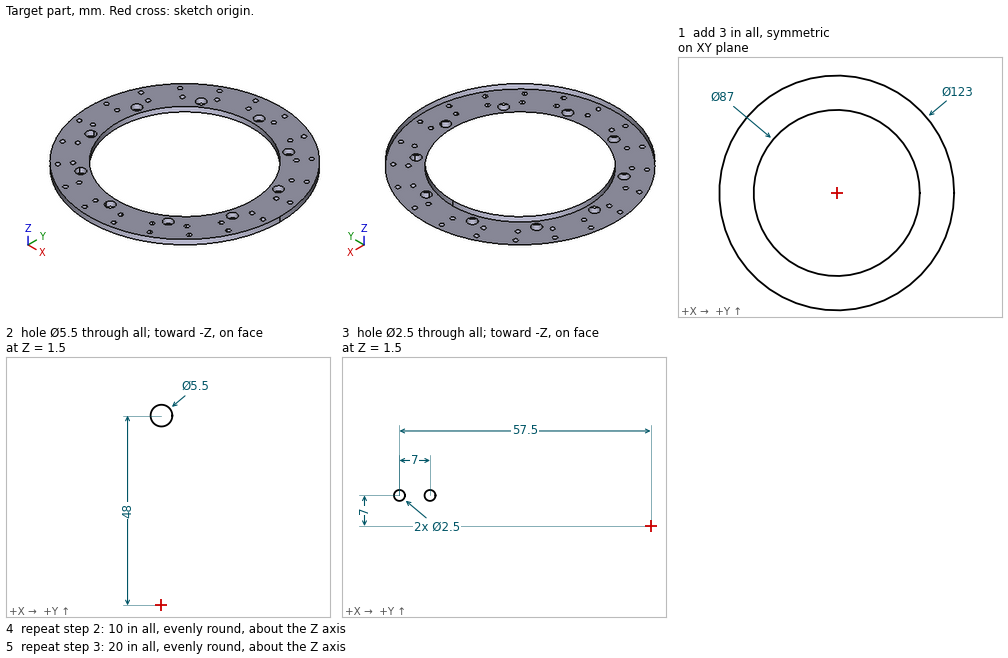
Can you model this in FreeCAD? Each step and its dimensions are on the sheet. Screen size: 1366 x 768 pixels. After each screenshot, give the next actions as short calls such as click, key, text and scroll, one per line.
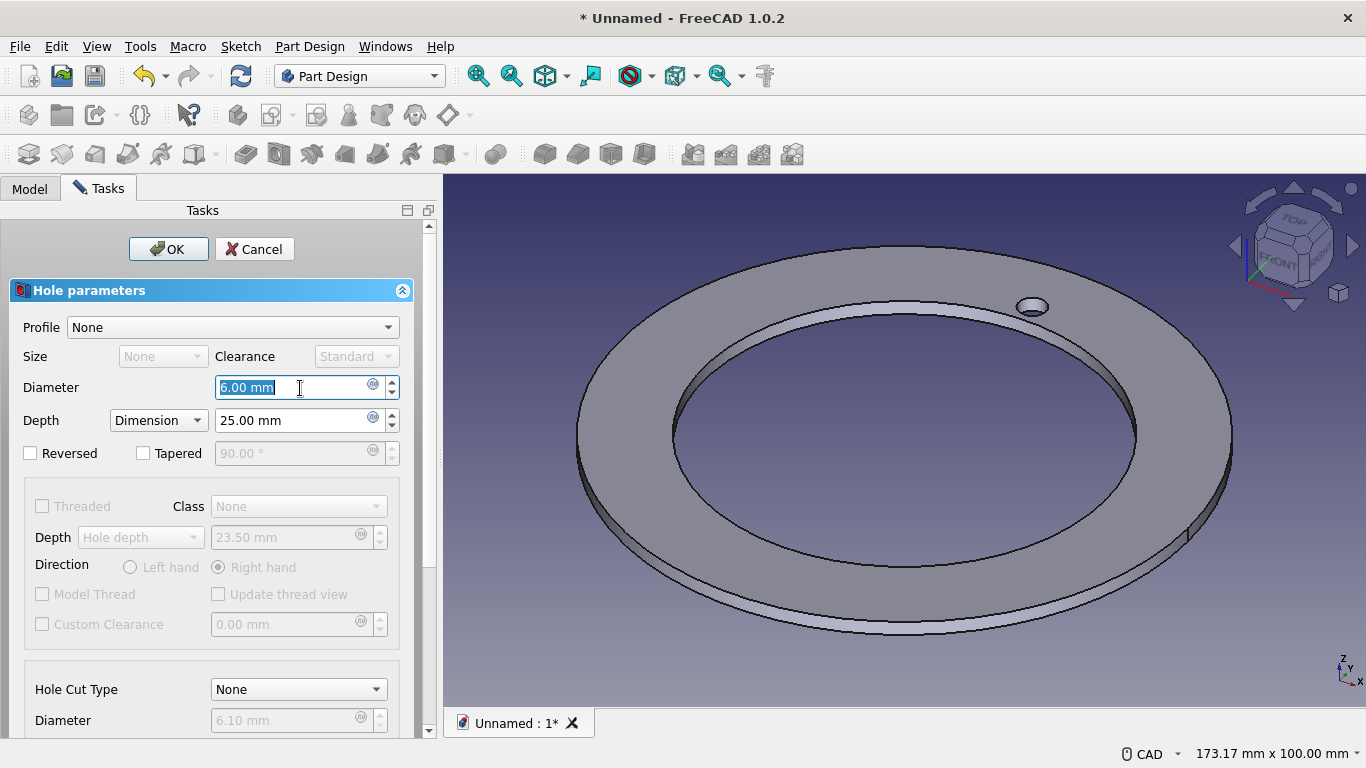
text(5.5)
key(Tab)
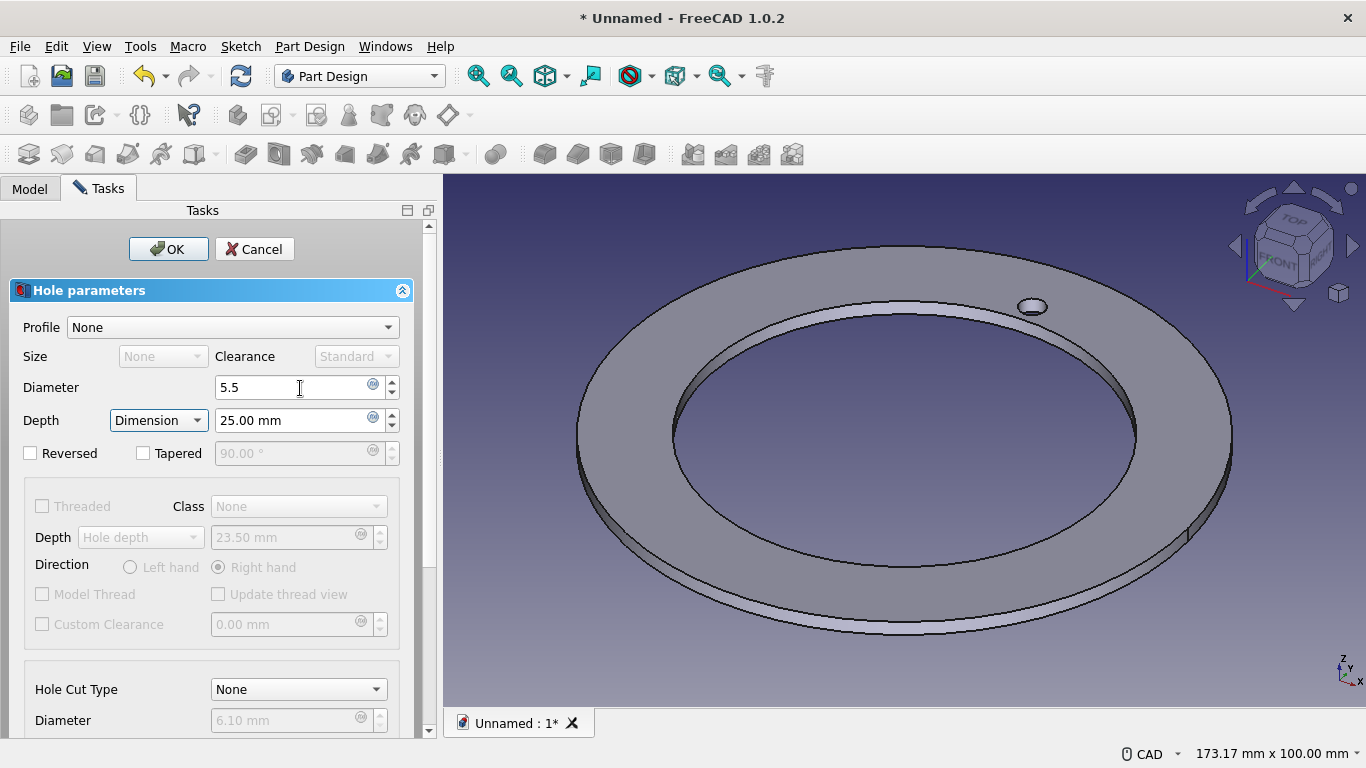
click(160, 420)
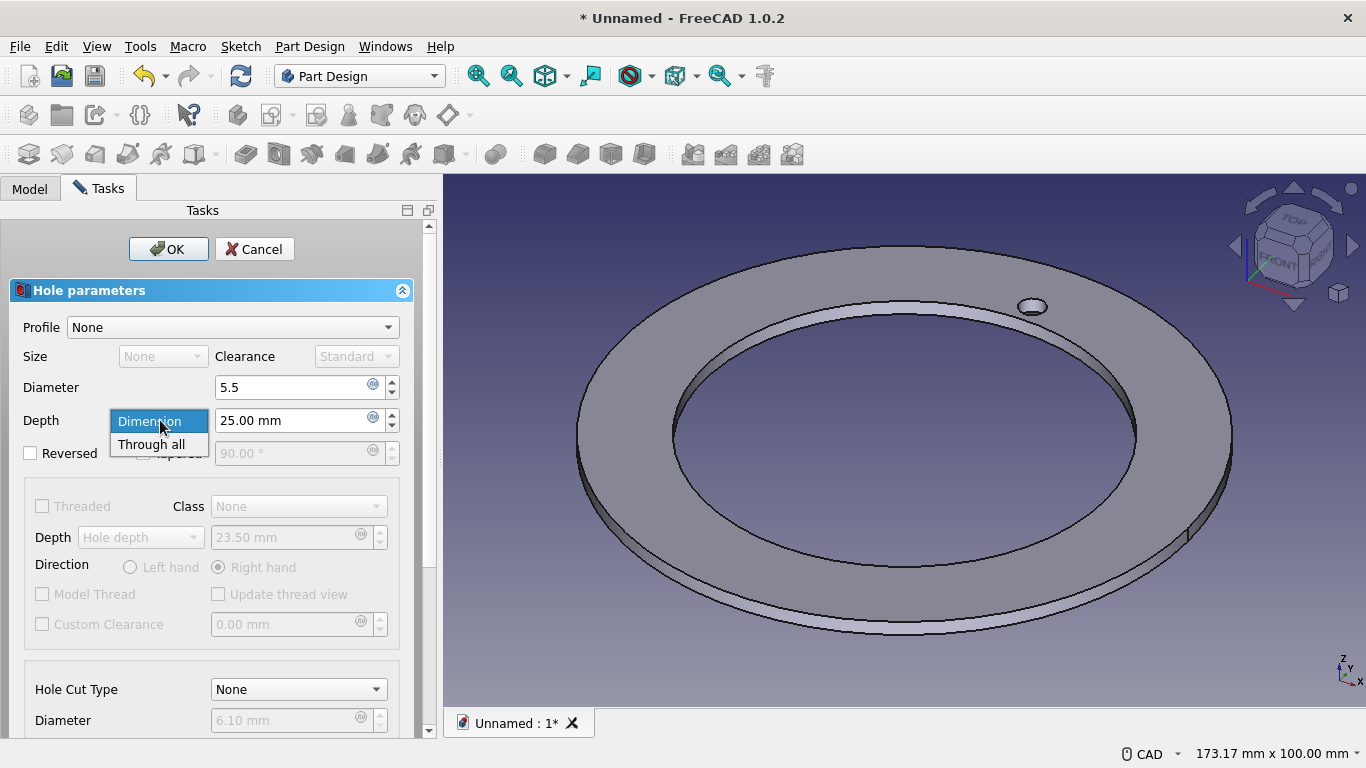
click(158, 444)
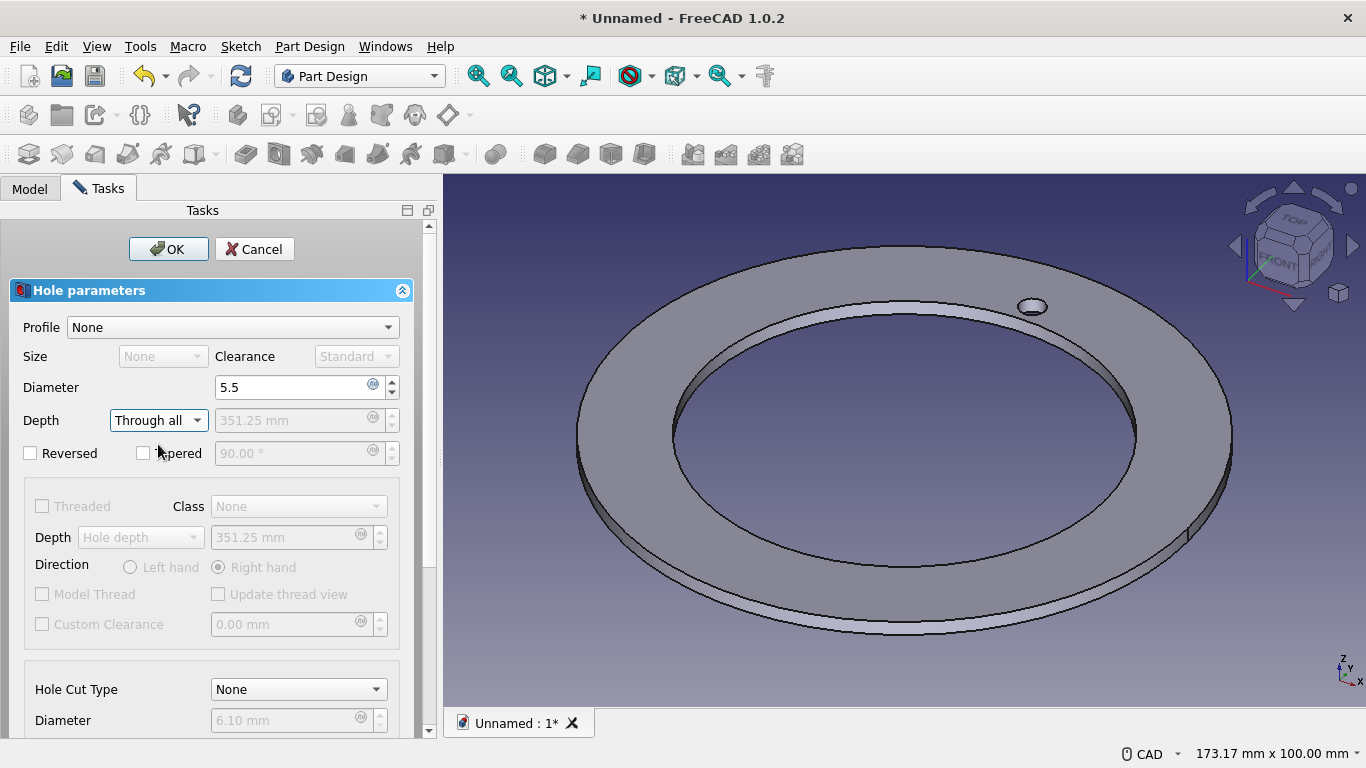
click(169, 249)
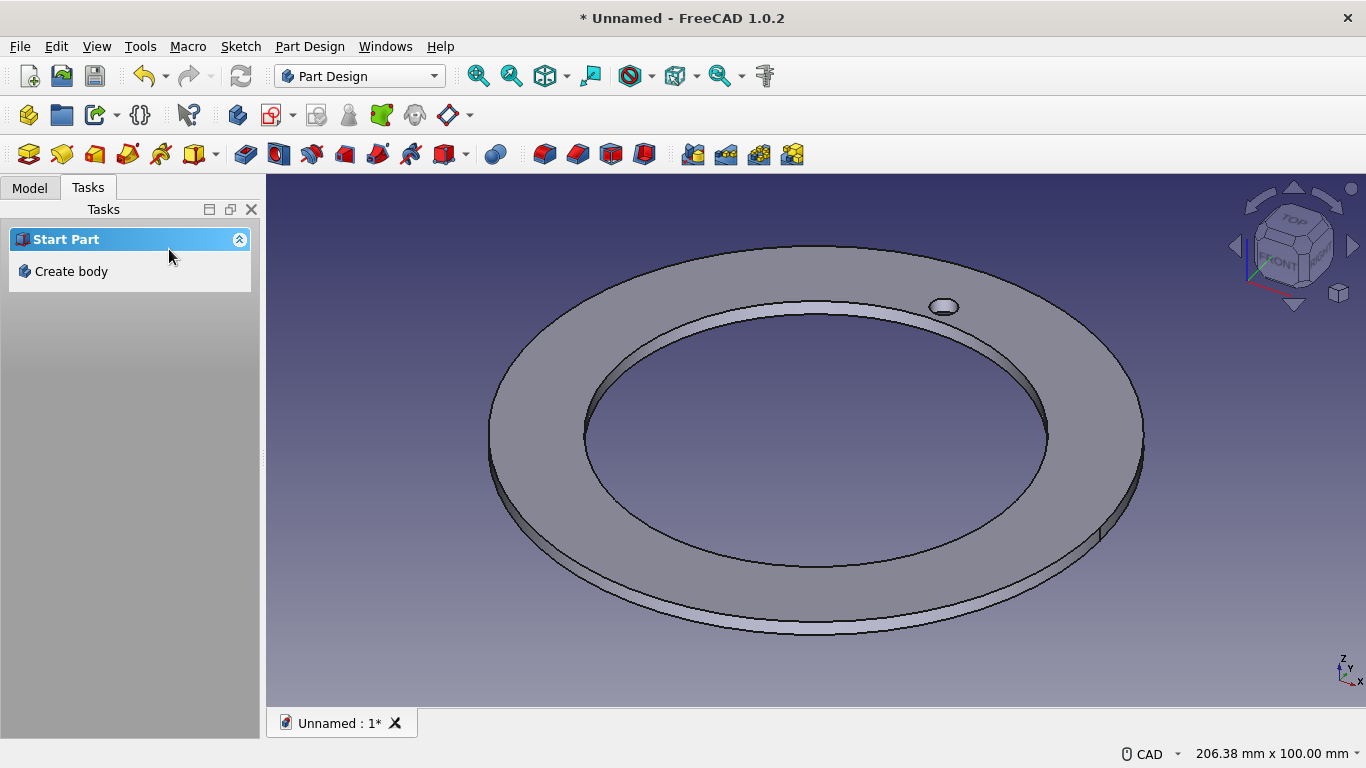
click(1059, 514)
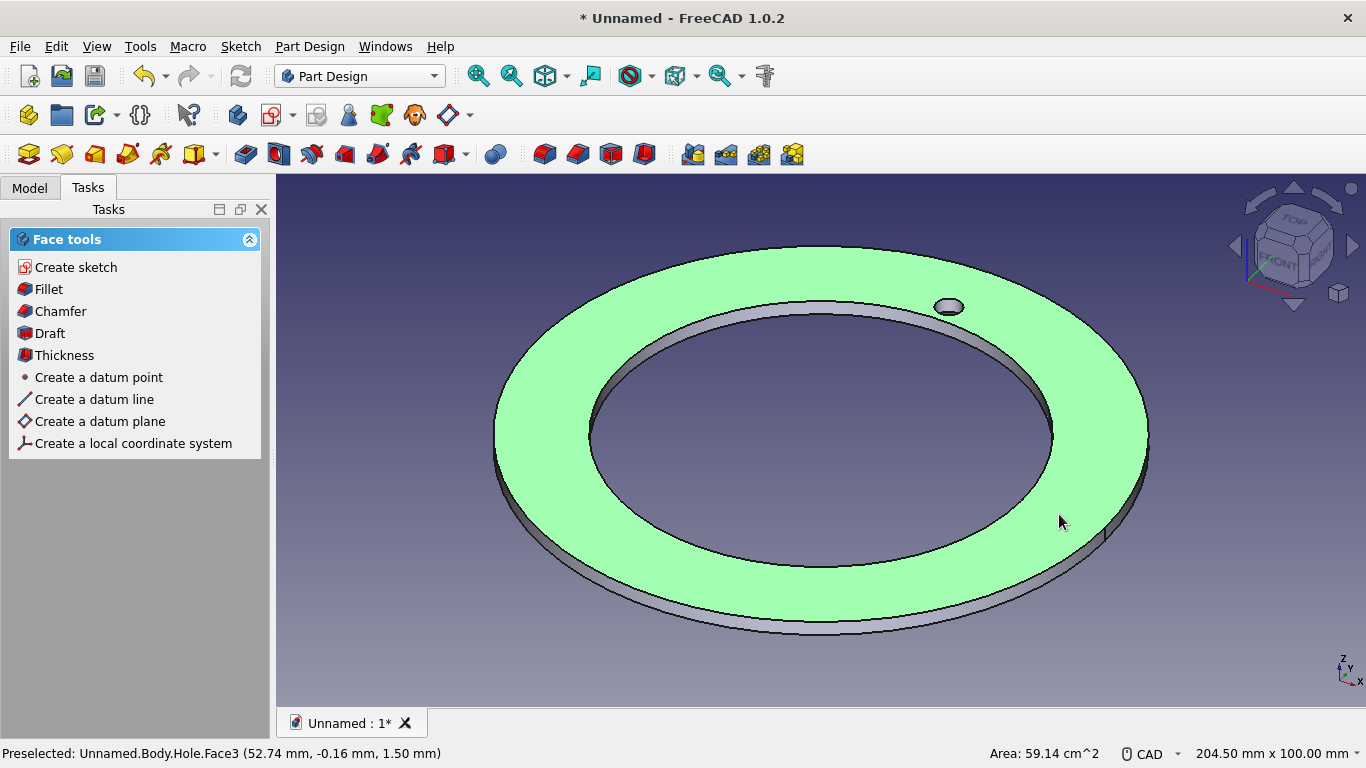
click(270, 116)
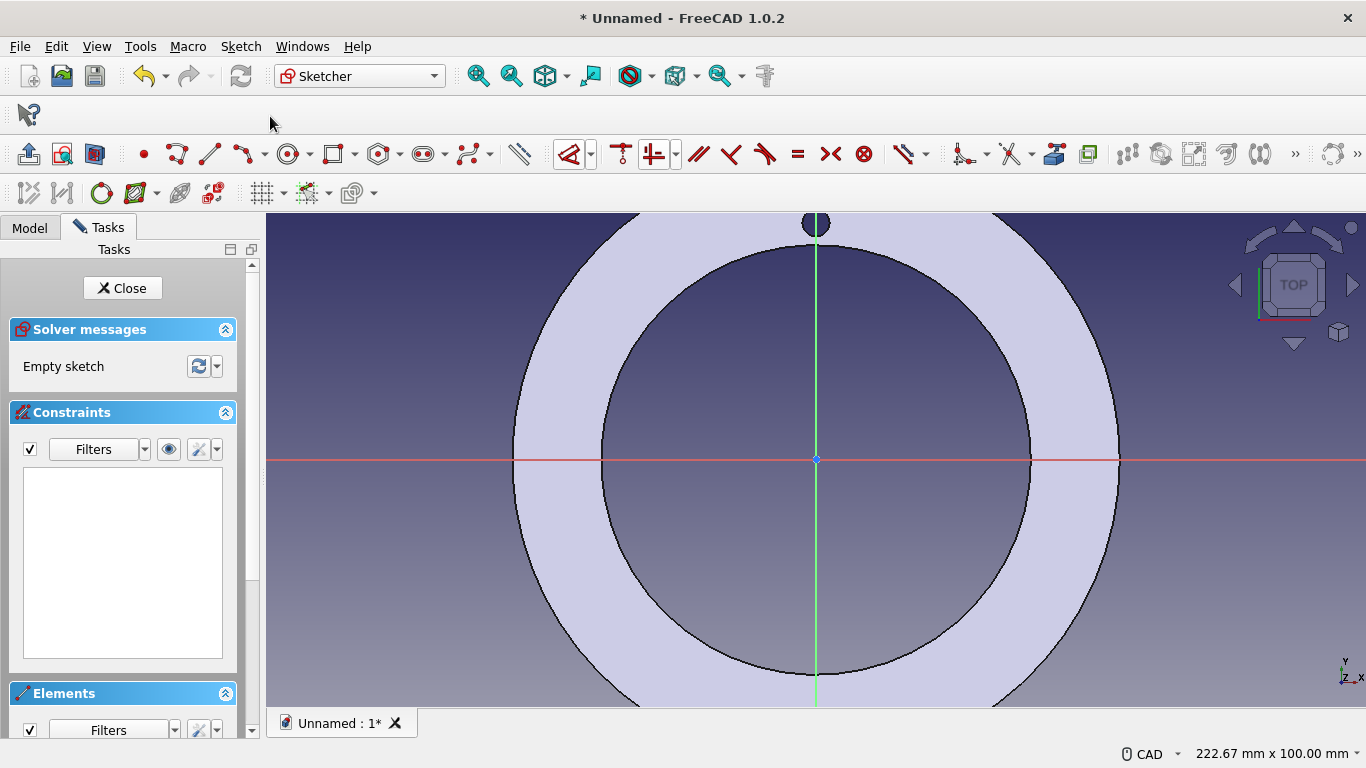
scroll(533, 423, up, 13)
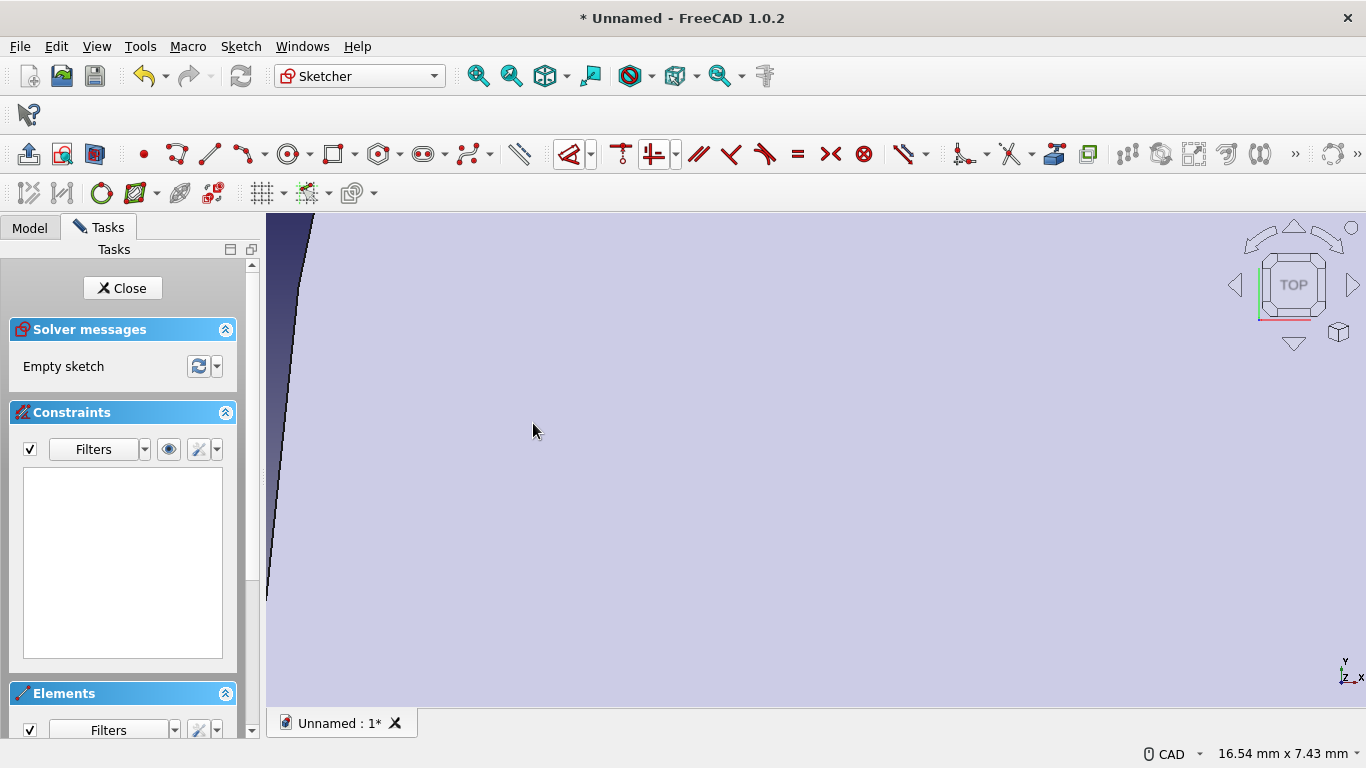
key(g)
key(c)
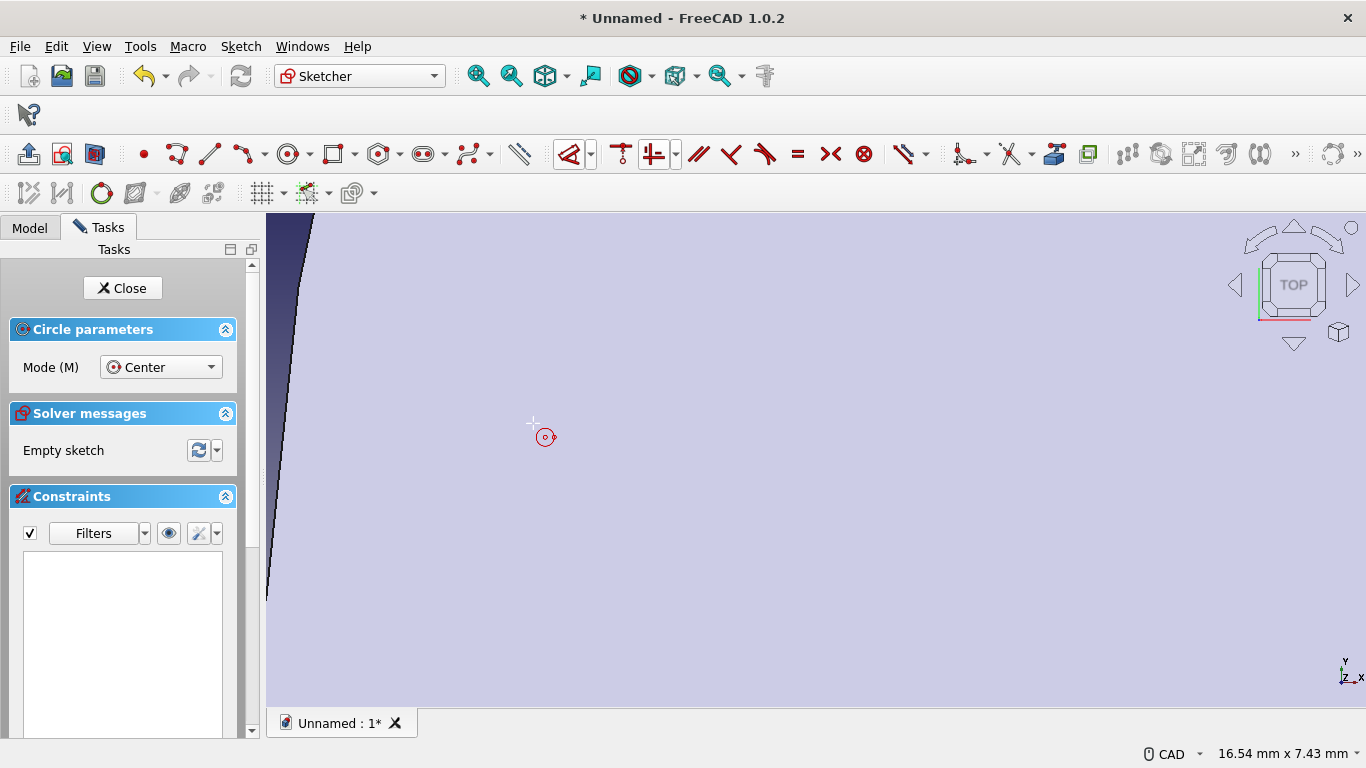
click(516, 450)
move(575, 391)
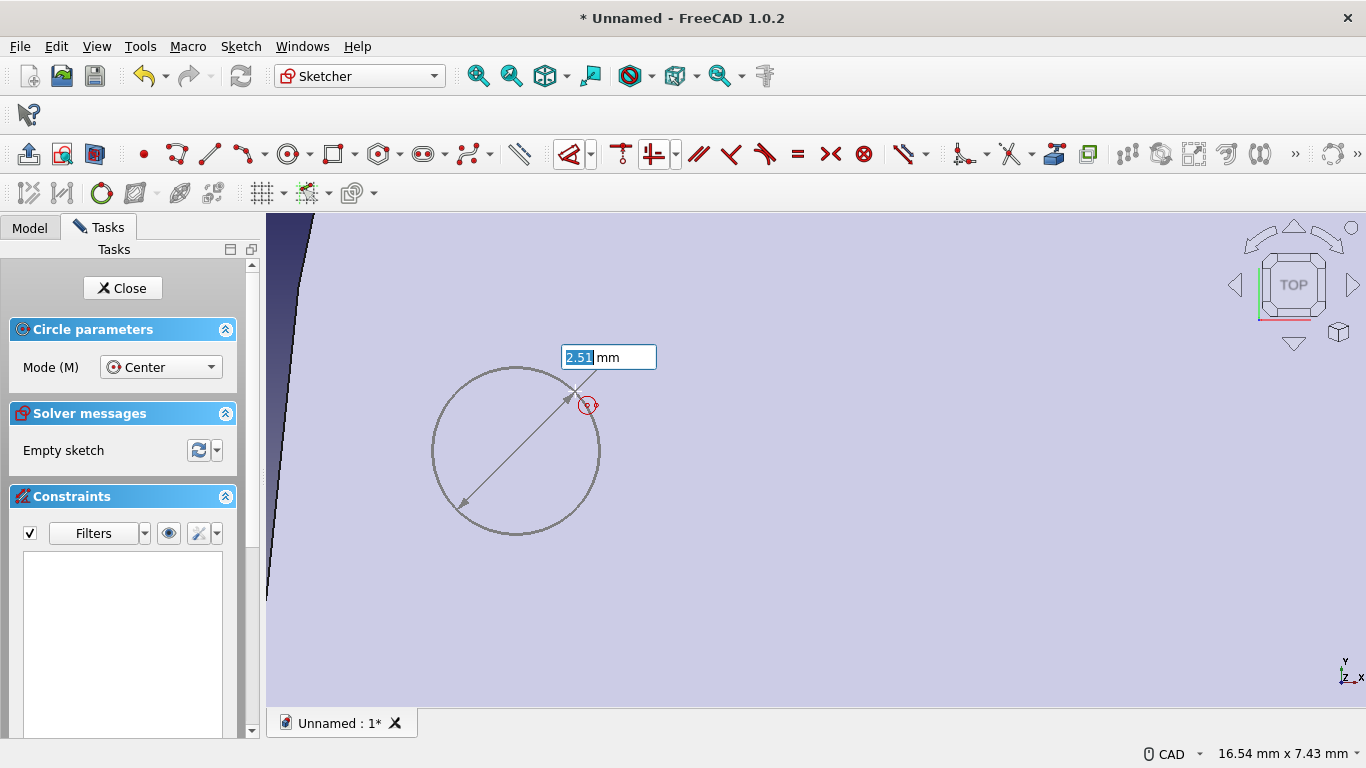
text(2.5)
key(Return)